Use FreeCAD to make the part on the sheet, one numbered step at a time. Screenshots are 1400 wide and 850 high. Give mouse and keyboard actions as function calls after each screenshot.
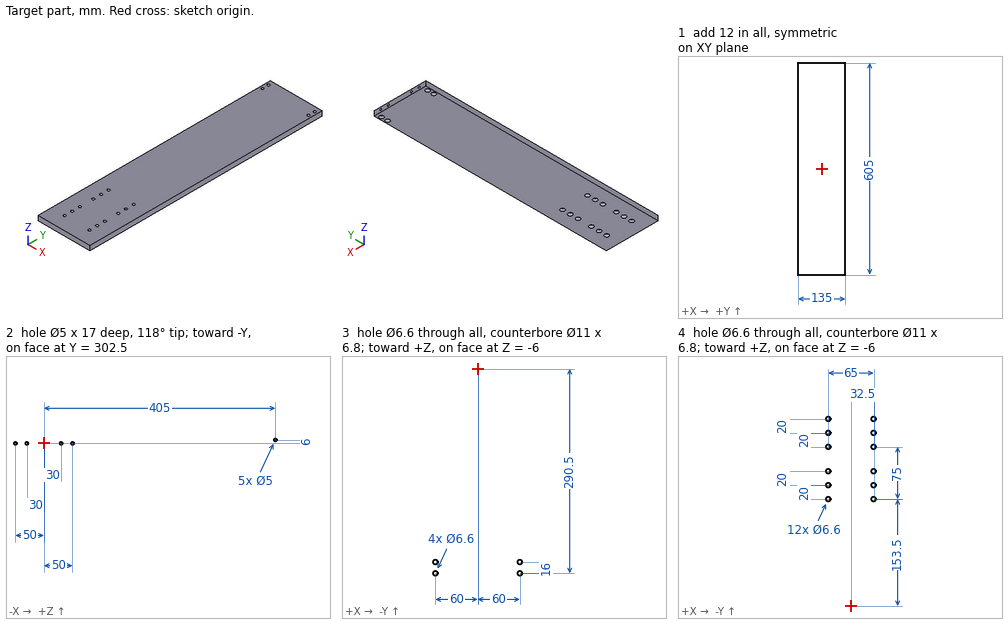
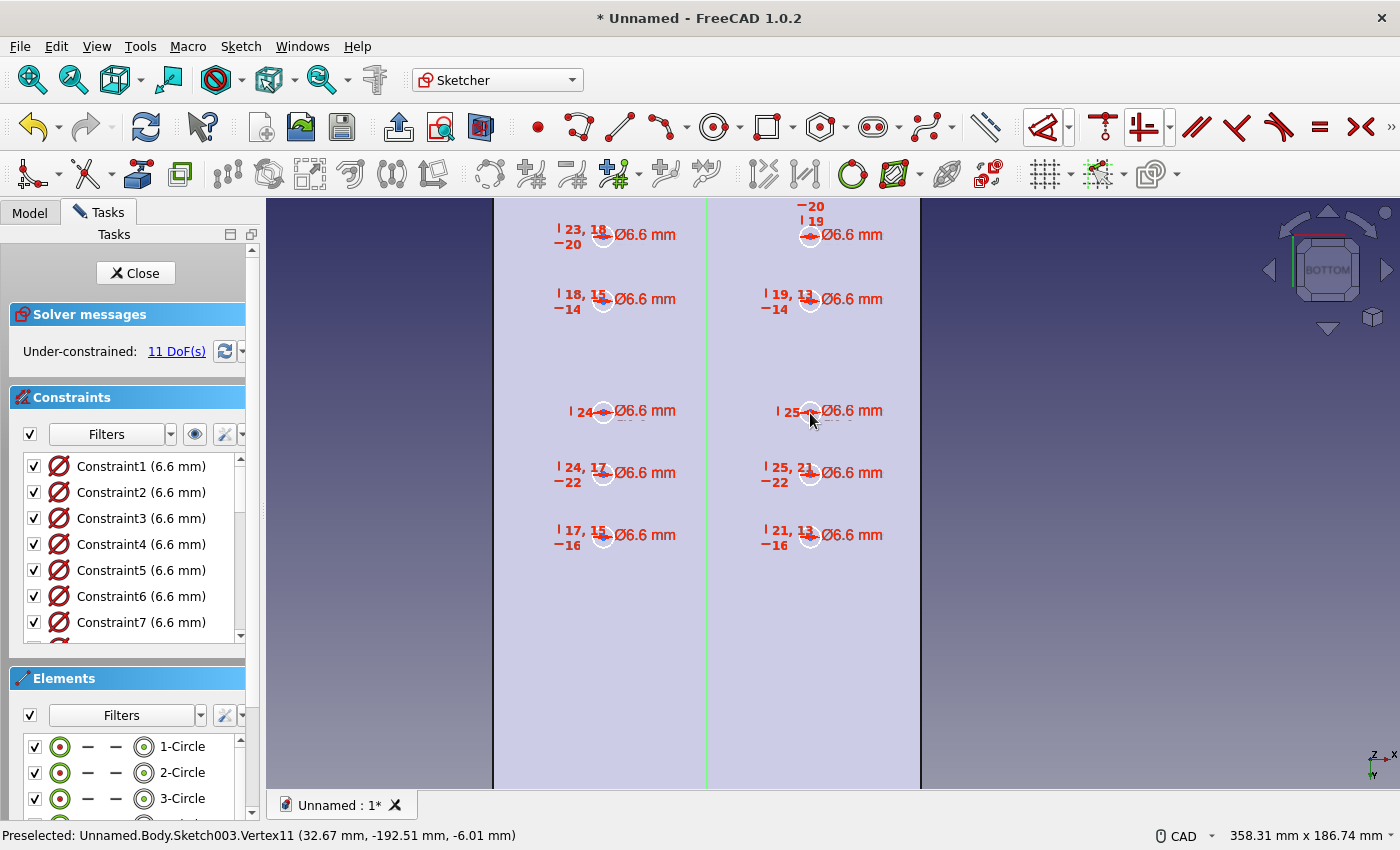
click(603, 413)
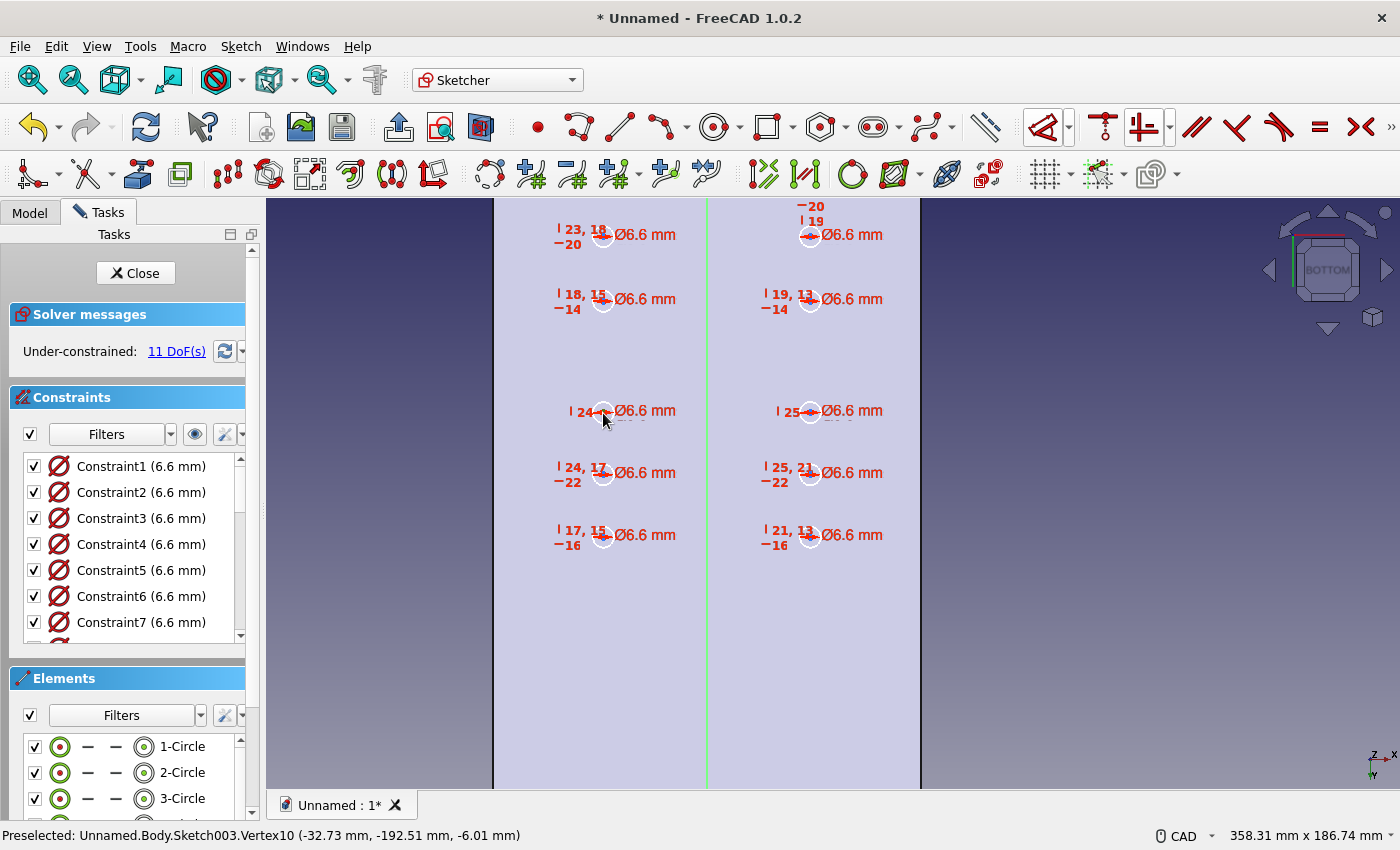
click(810, 413)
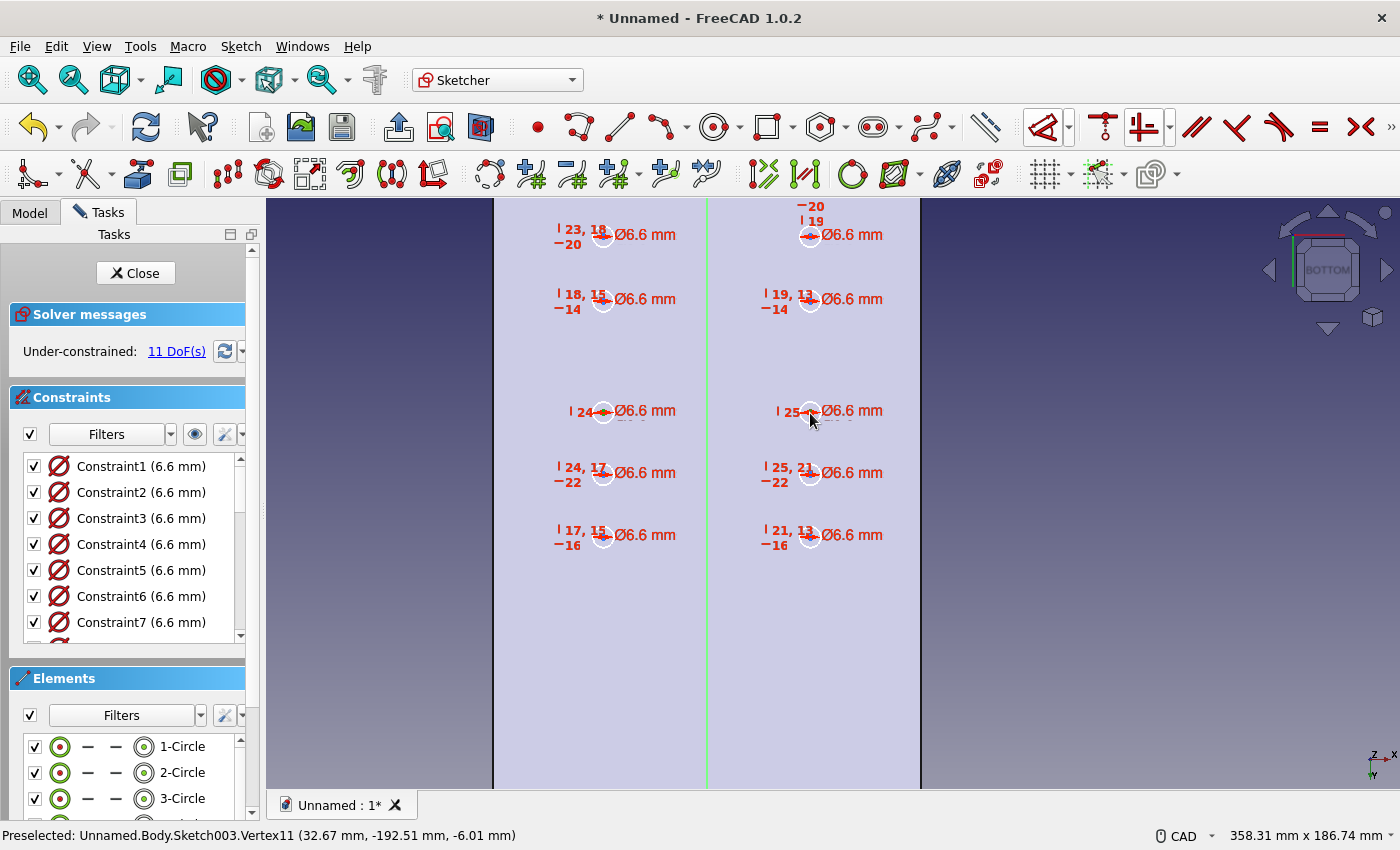
click(1170, 128)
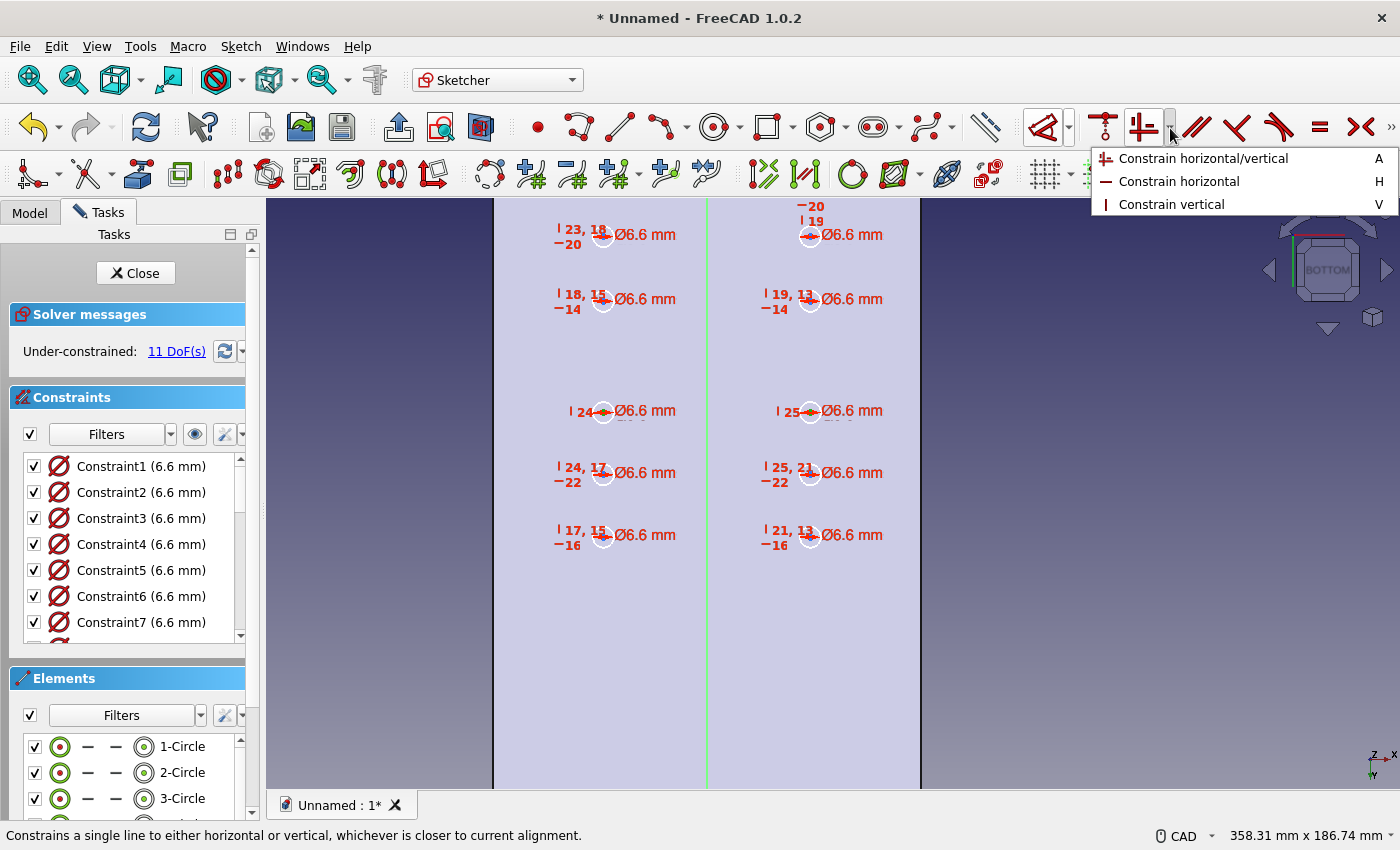
click(1245, 182)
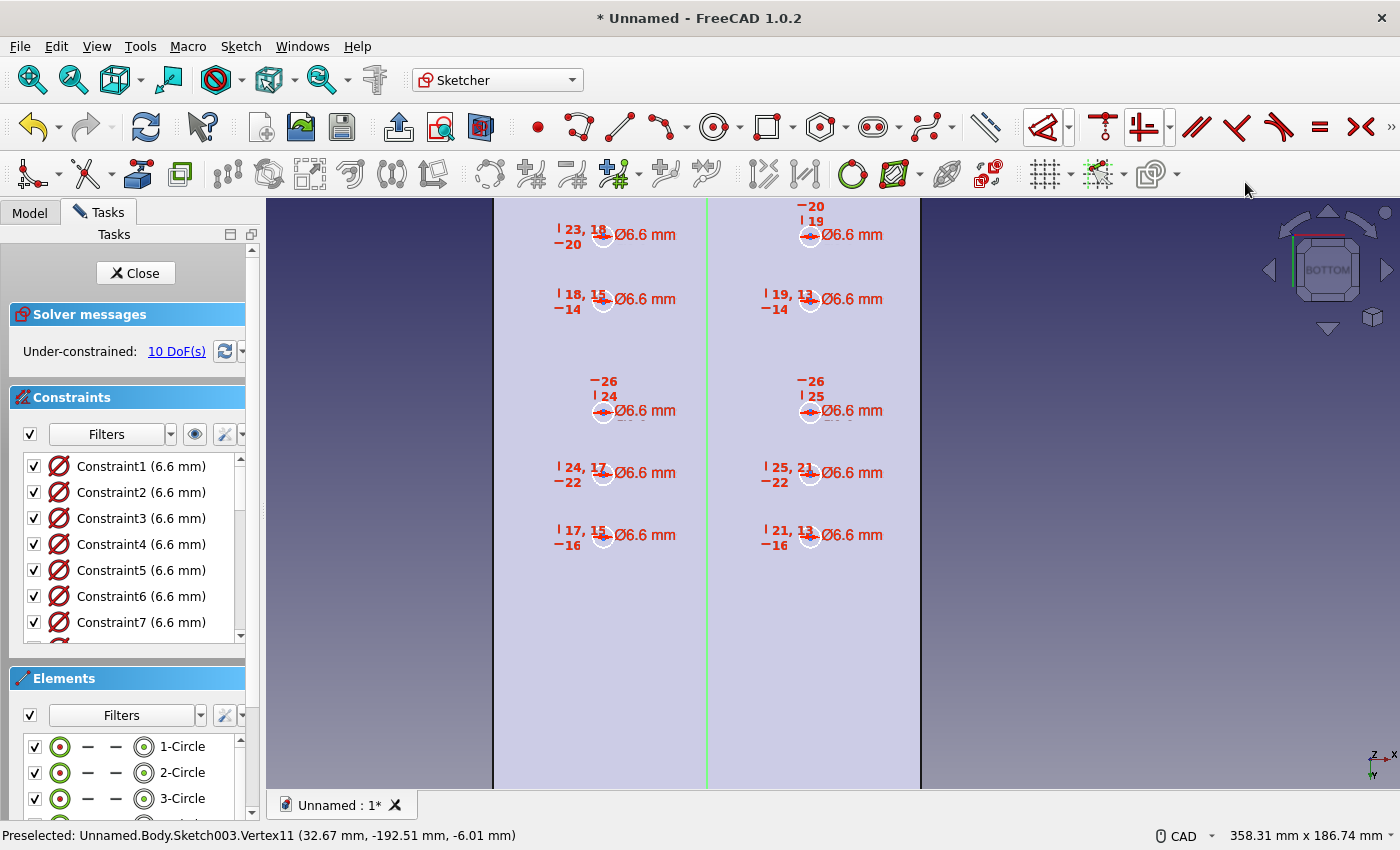
click(810, 237)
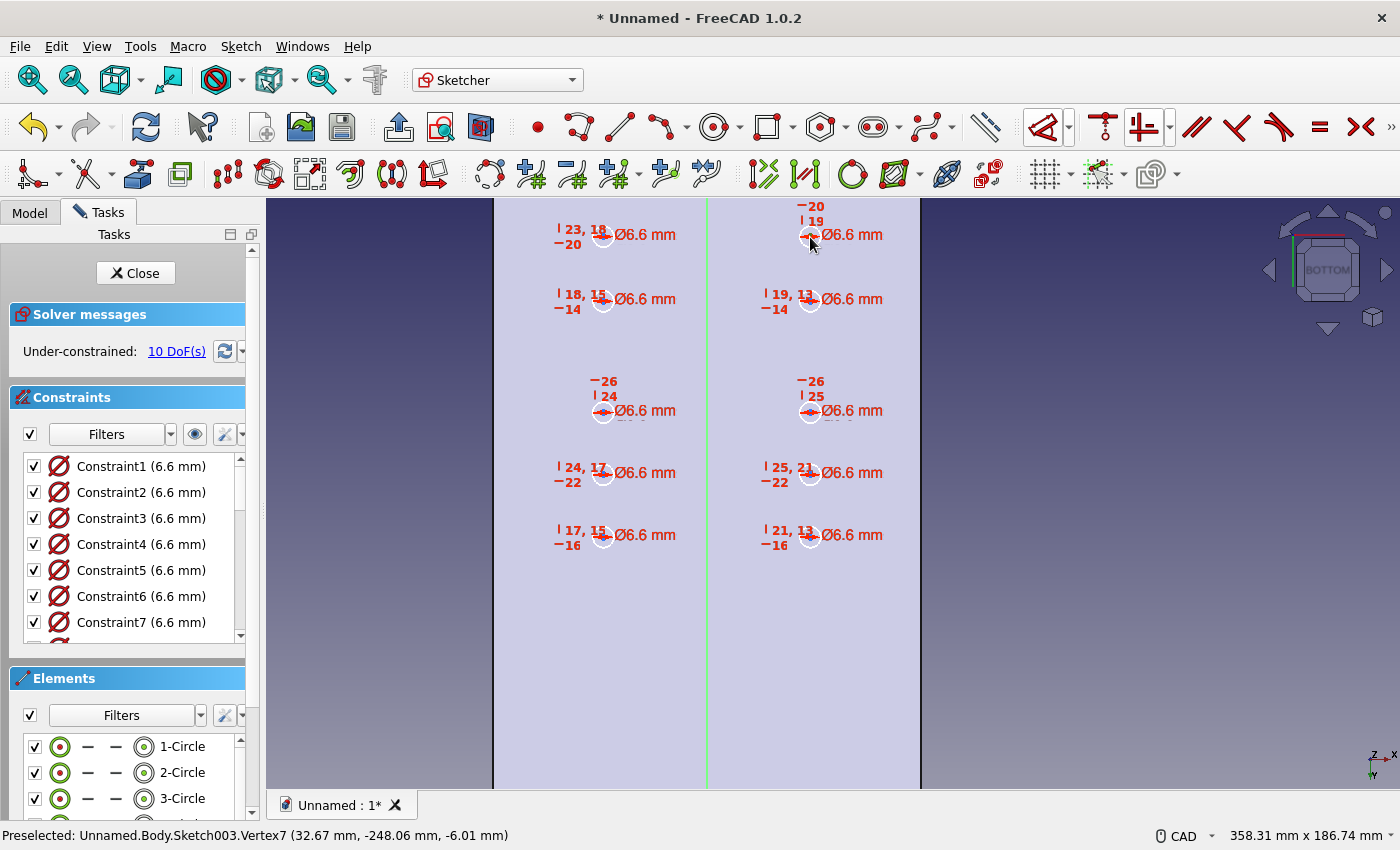
scroll(811, 413, down, 4)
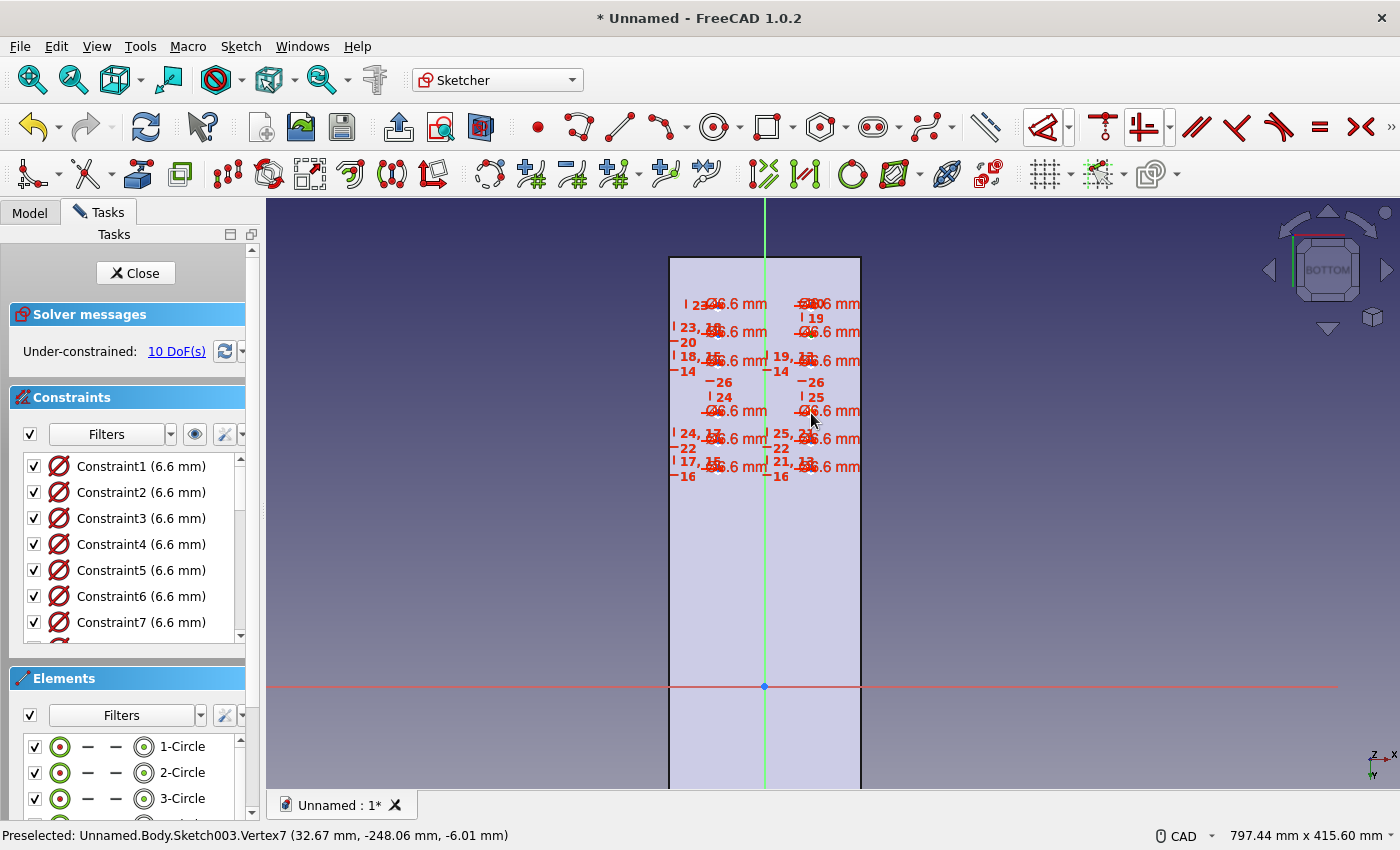
scroll(811, 306, up, 4)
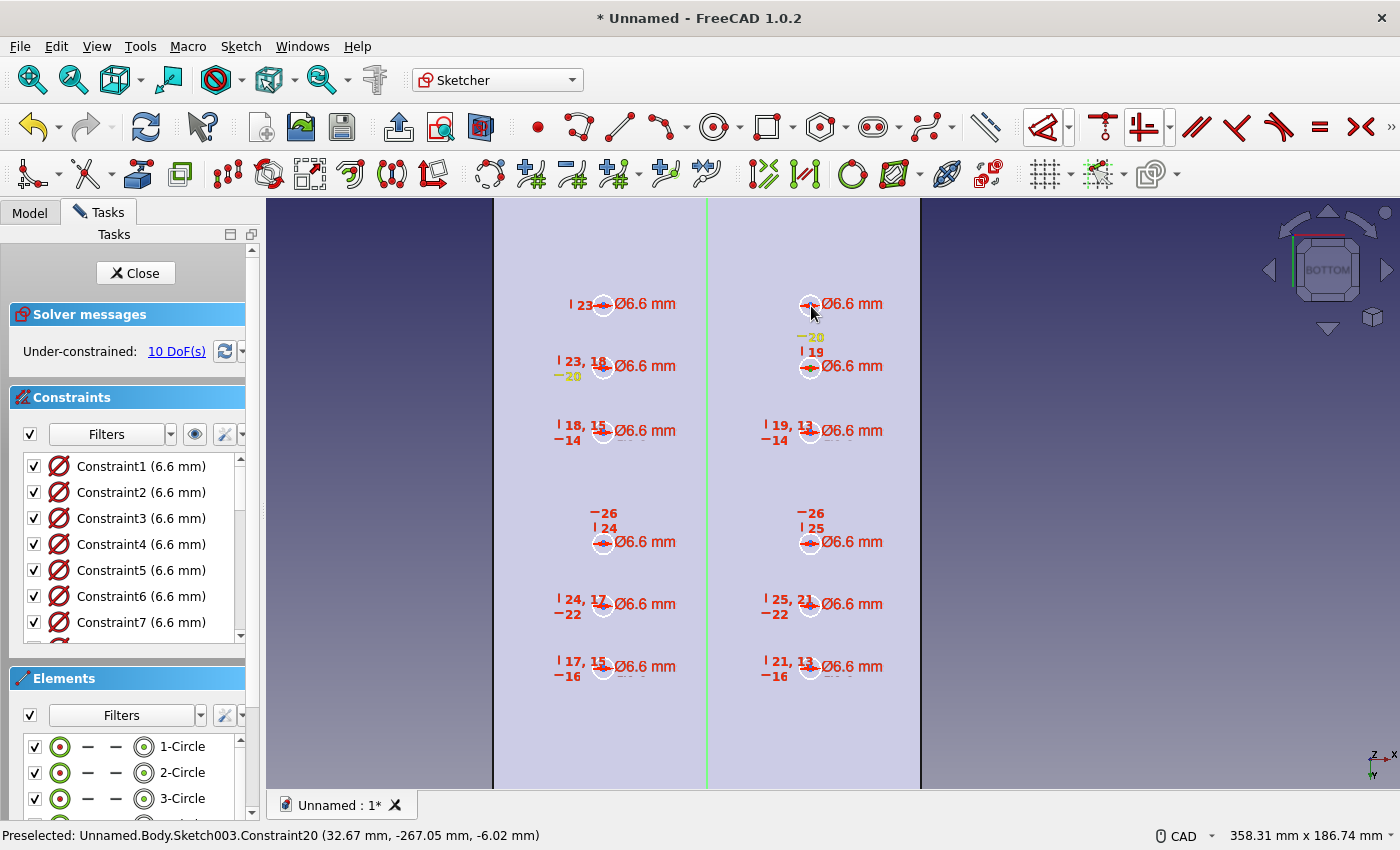
click(810, 306)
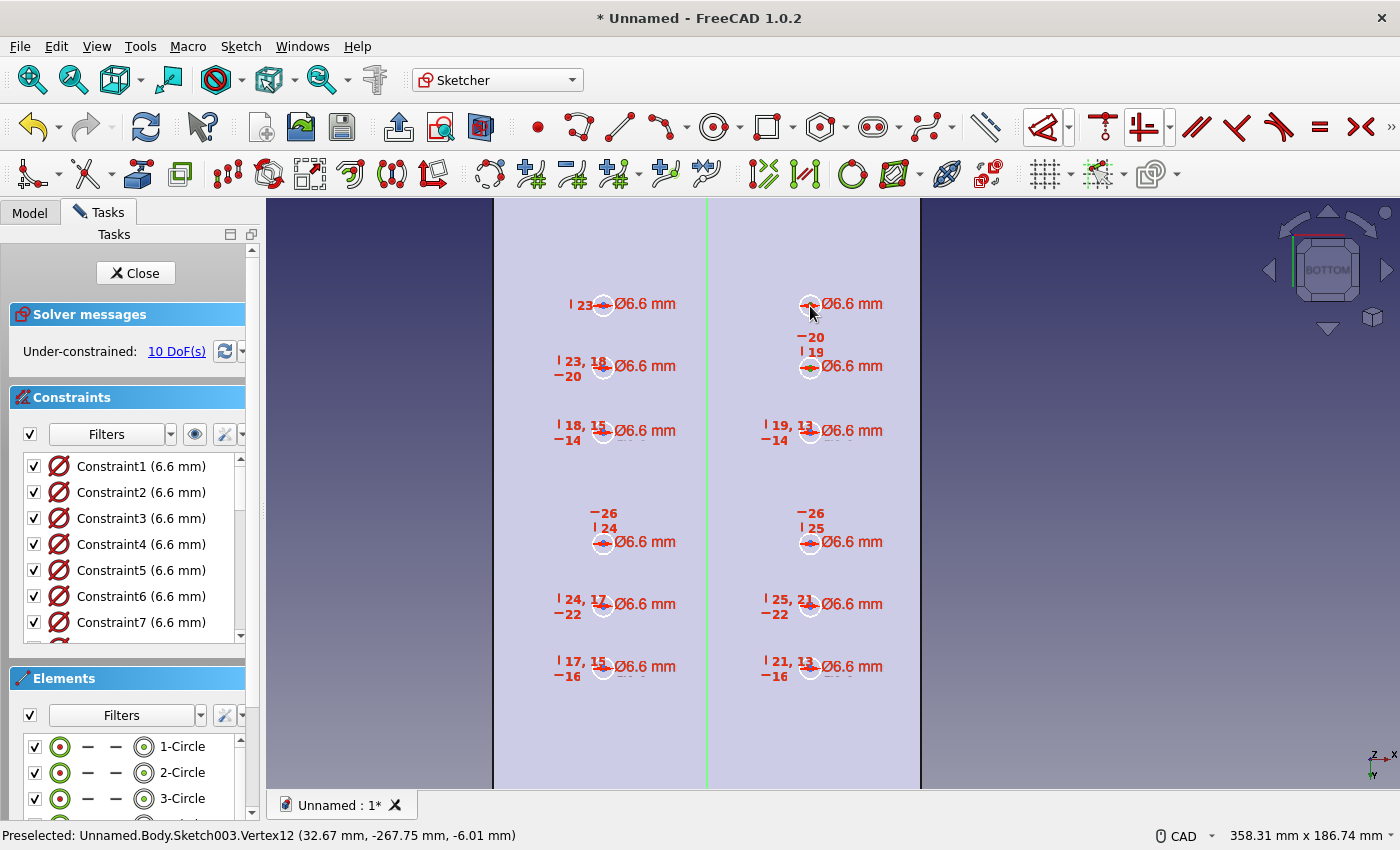
click(1170, 128)